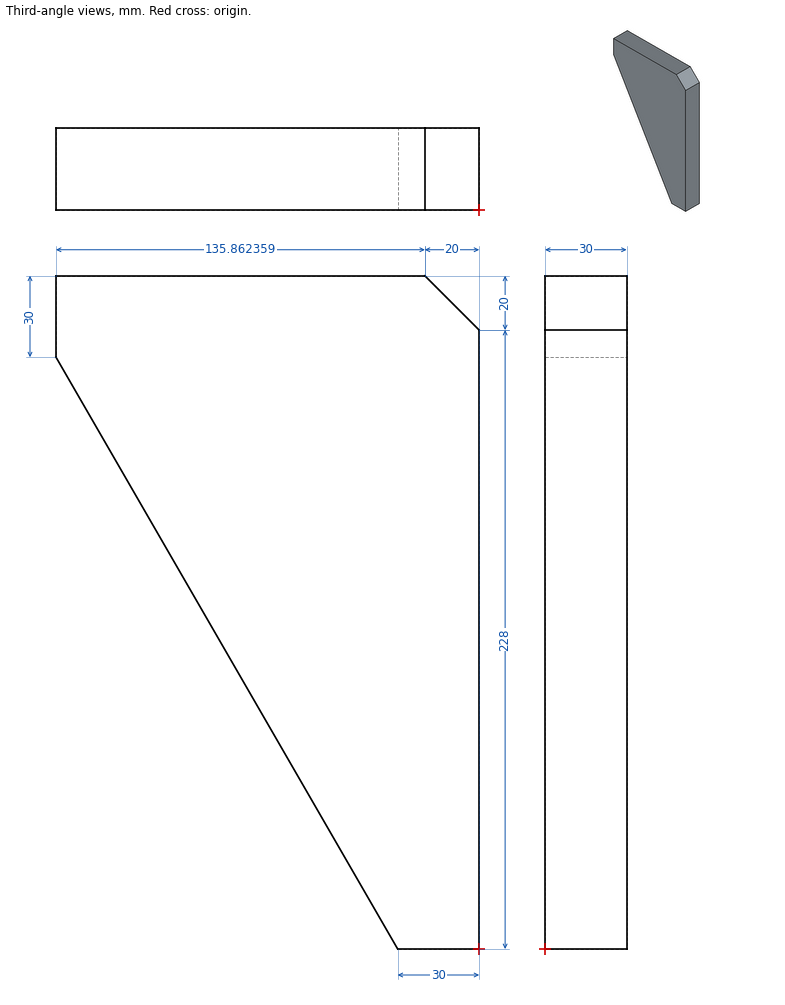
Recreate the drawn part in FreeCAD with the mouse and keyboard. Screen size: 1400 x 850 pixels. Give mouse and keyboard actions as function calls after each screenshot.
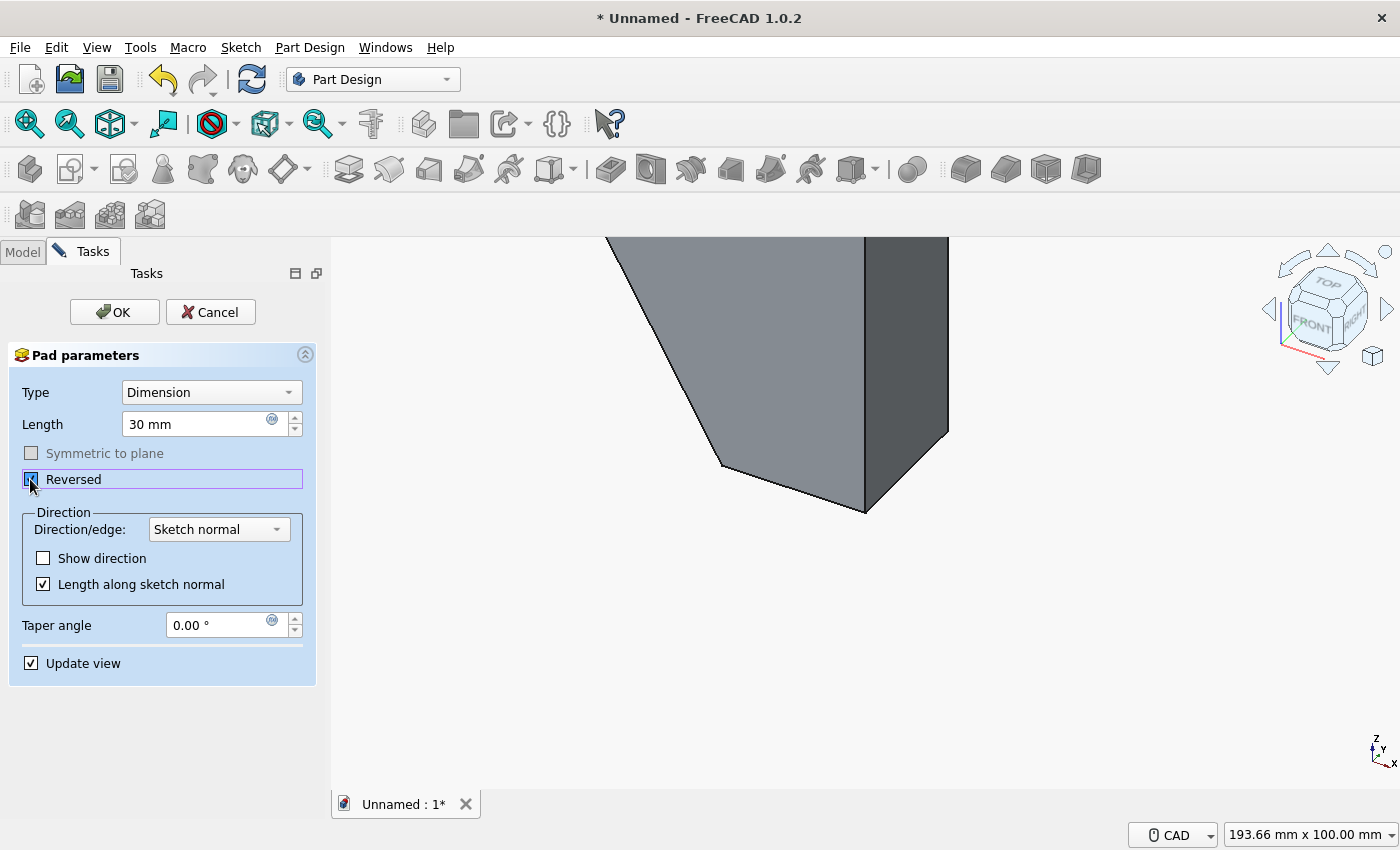
click(115, 312)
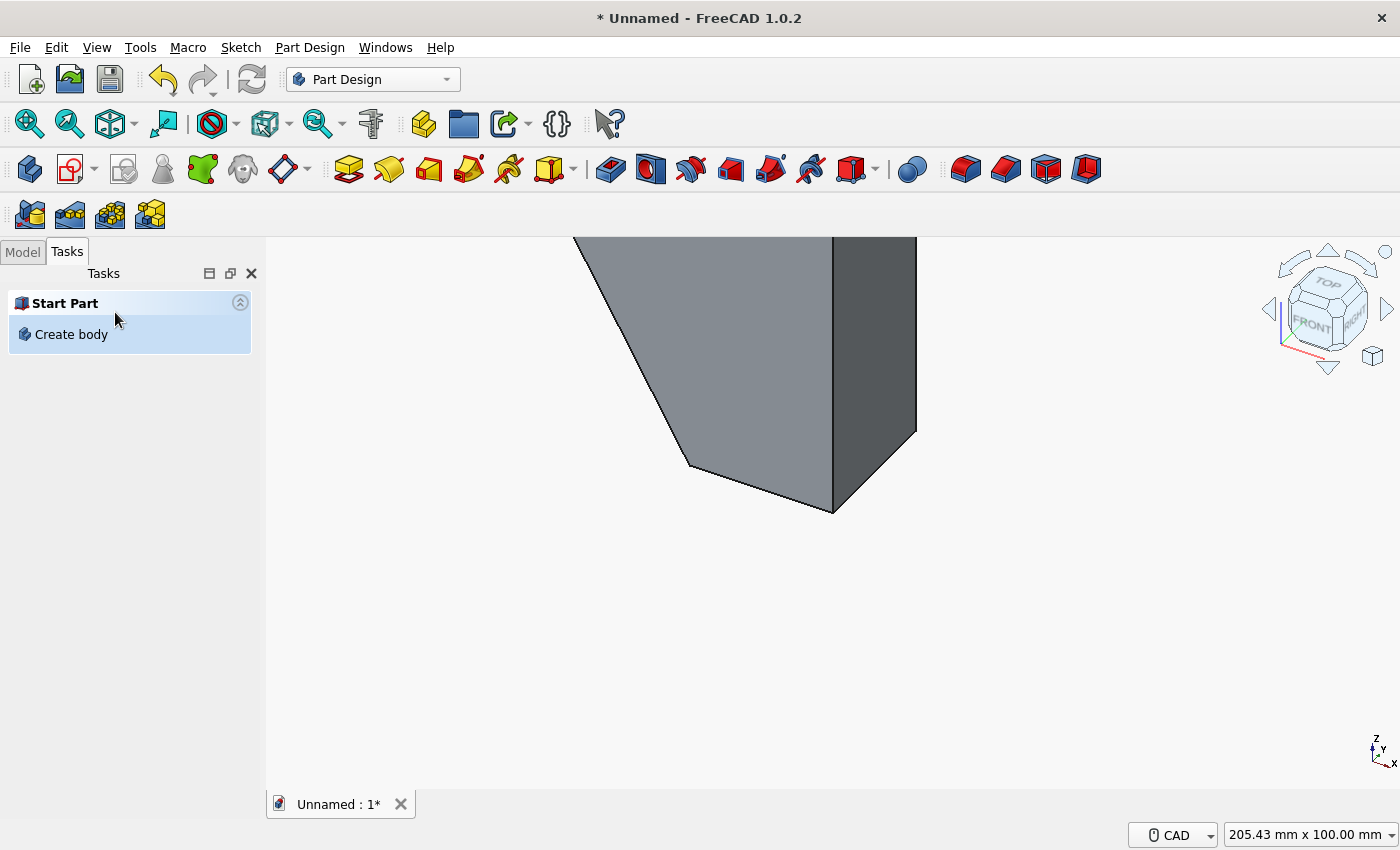
key(0)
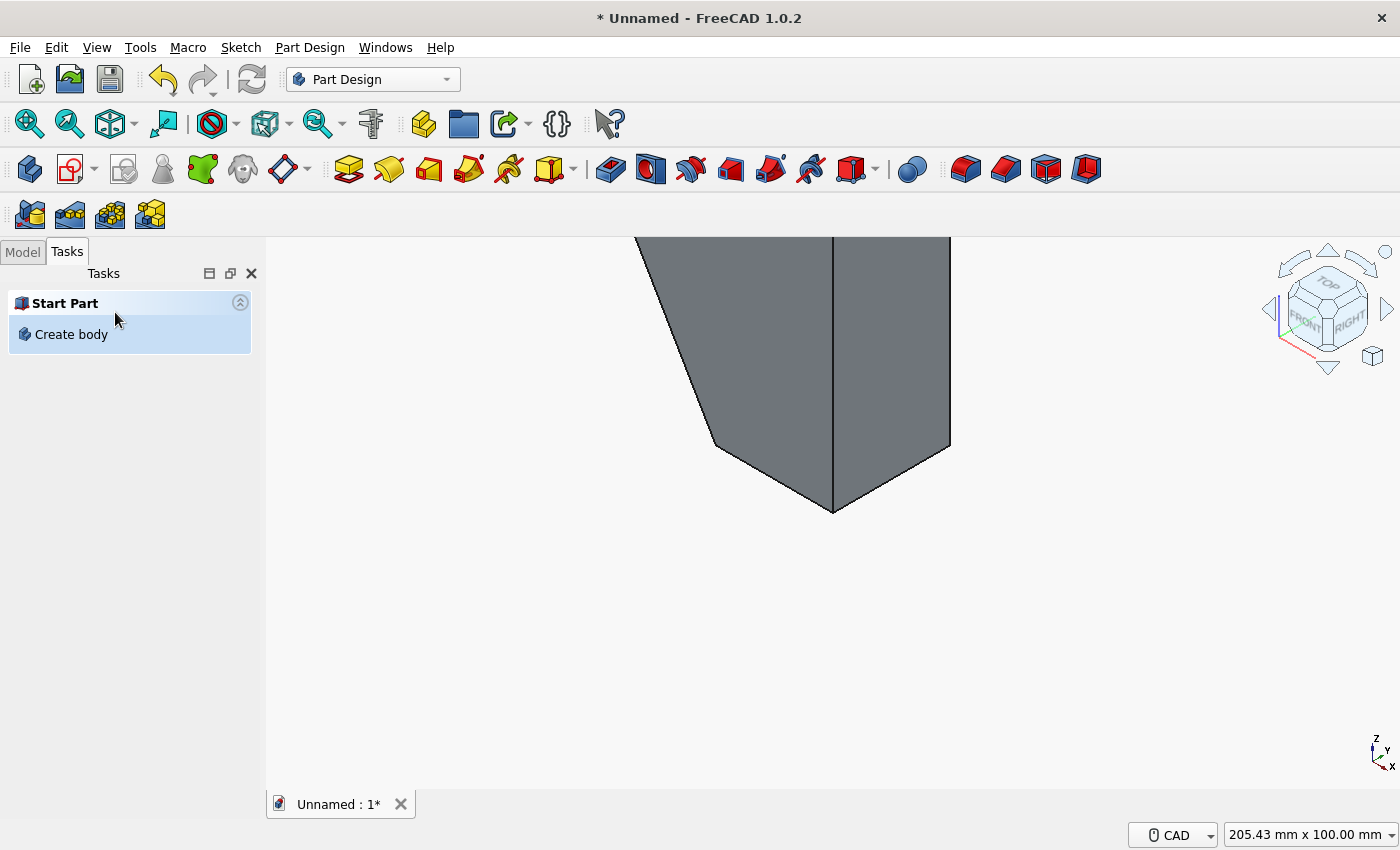
click(30, 124)